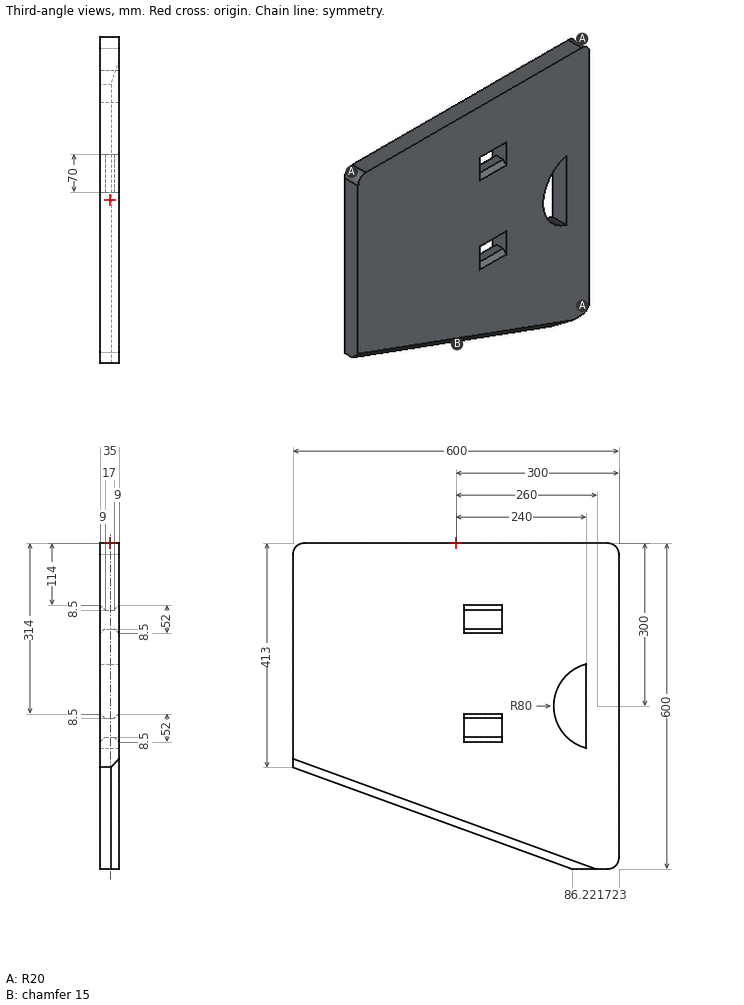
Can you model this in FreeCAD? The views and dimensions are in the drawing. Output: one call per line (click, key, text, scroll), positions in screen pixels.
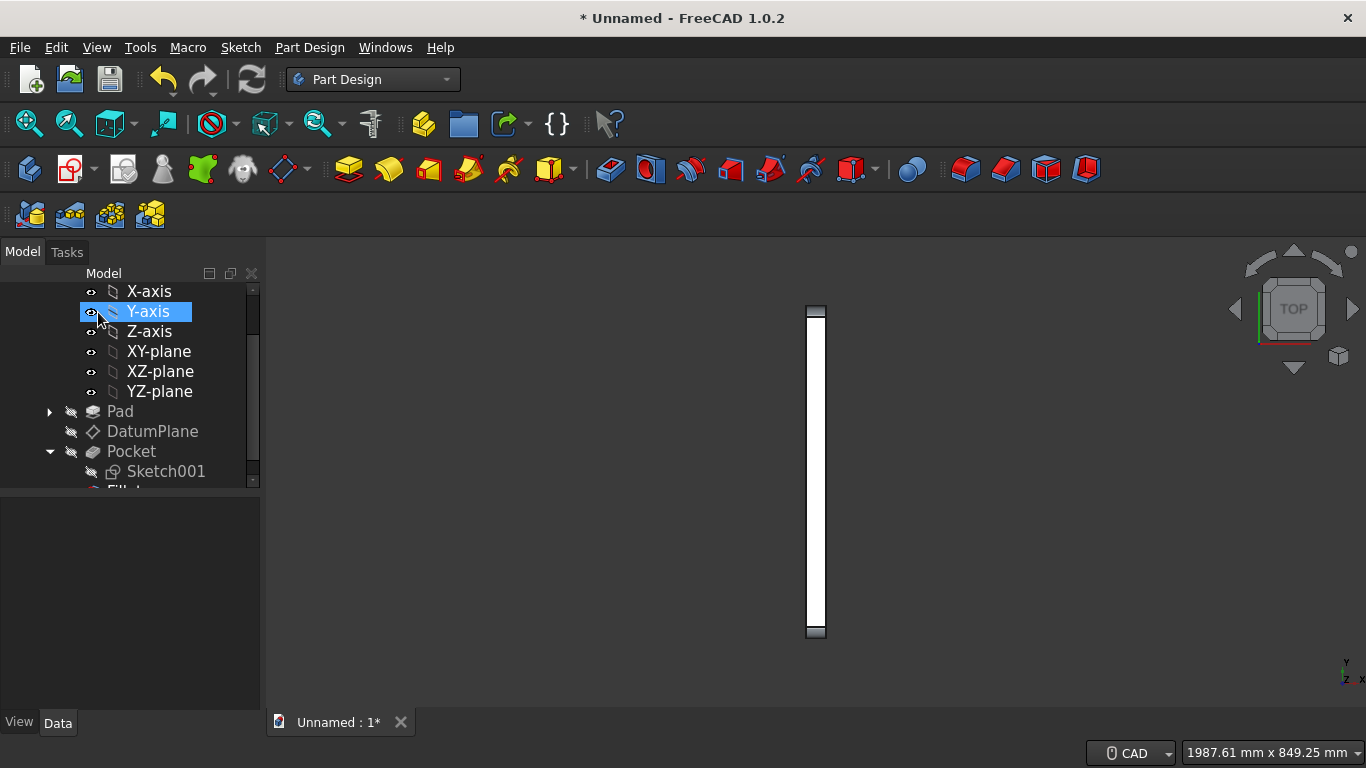
key(1)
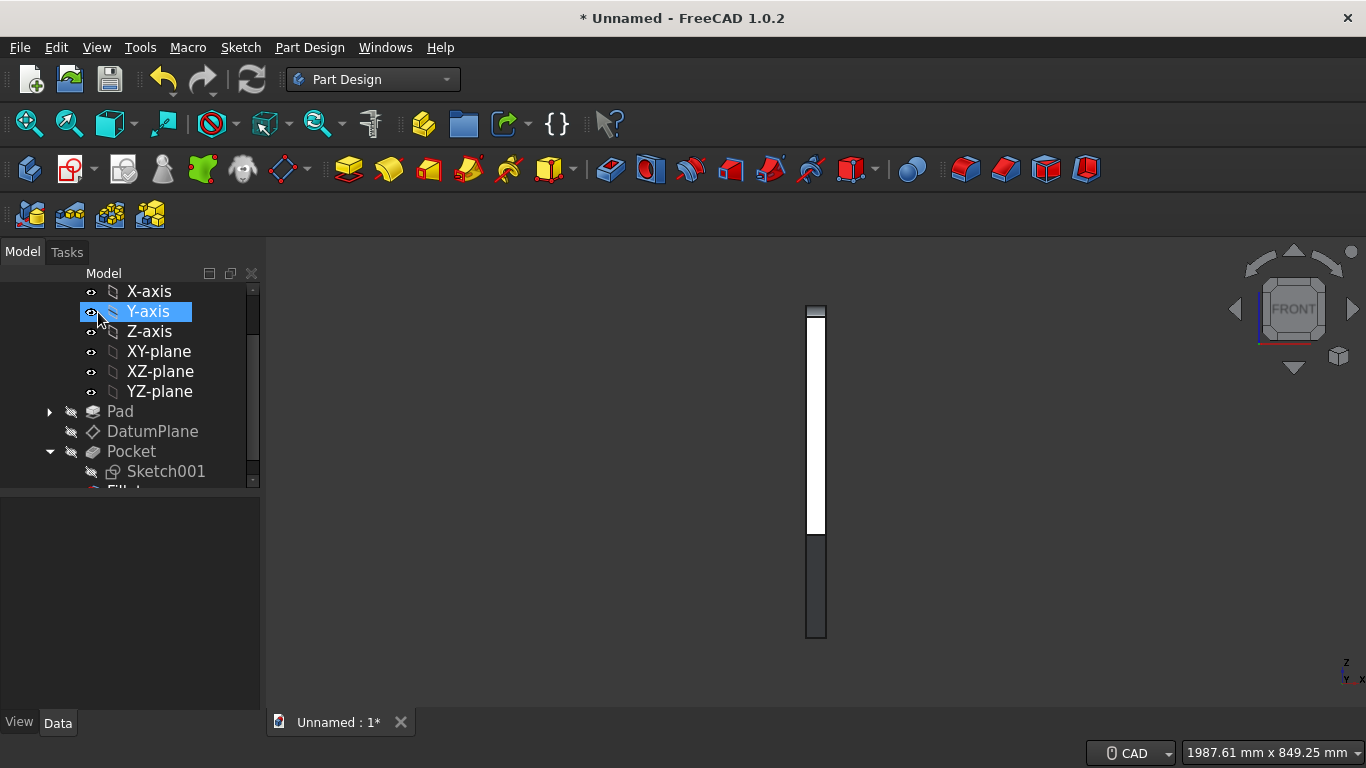
click(826, 585)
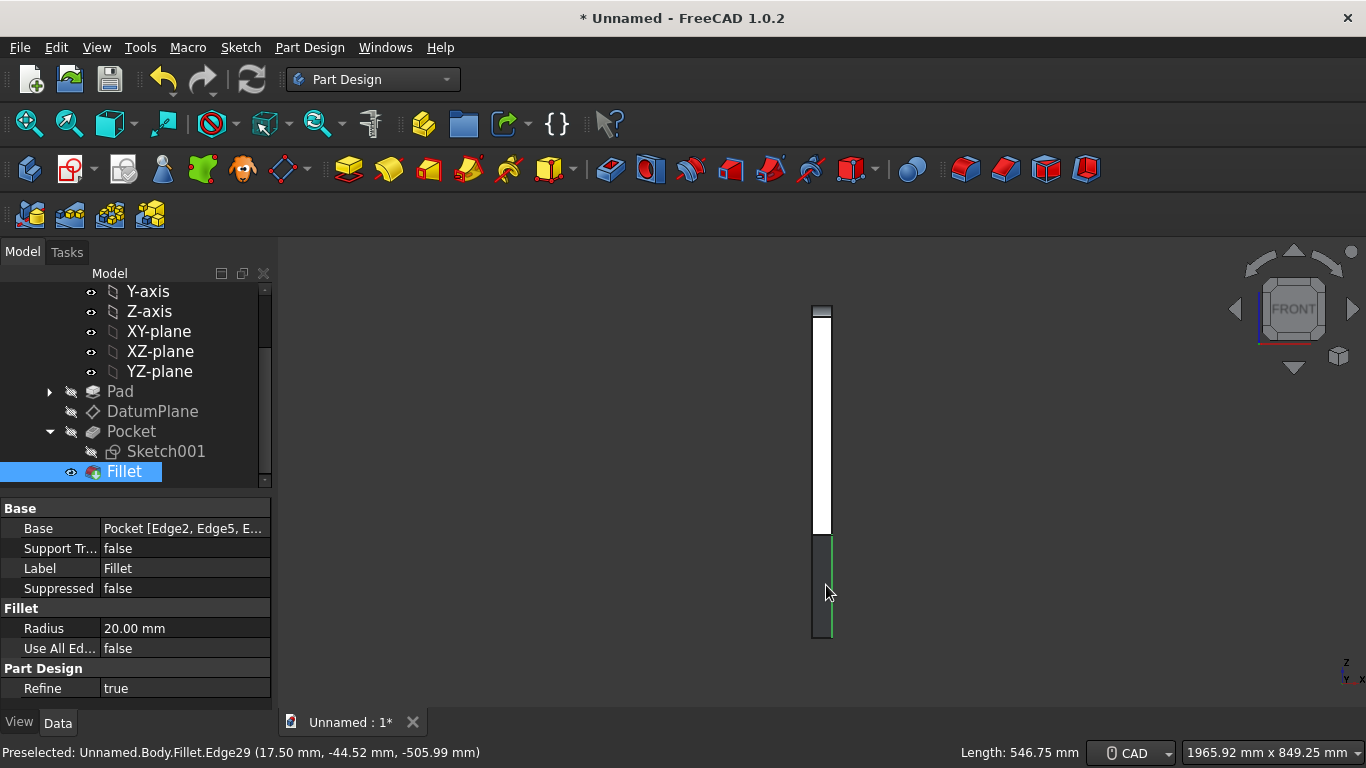
click(1006, 170)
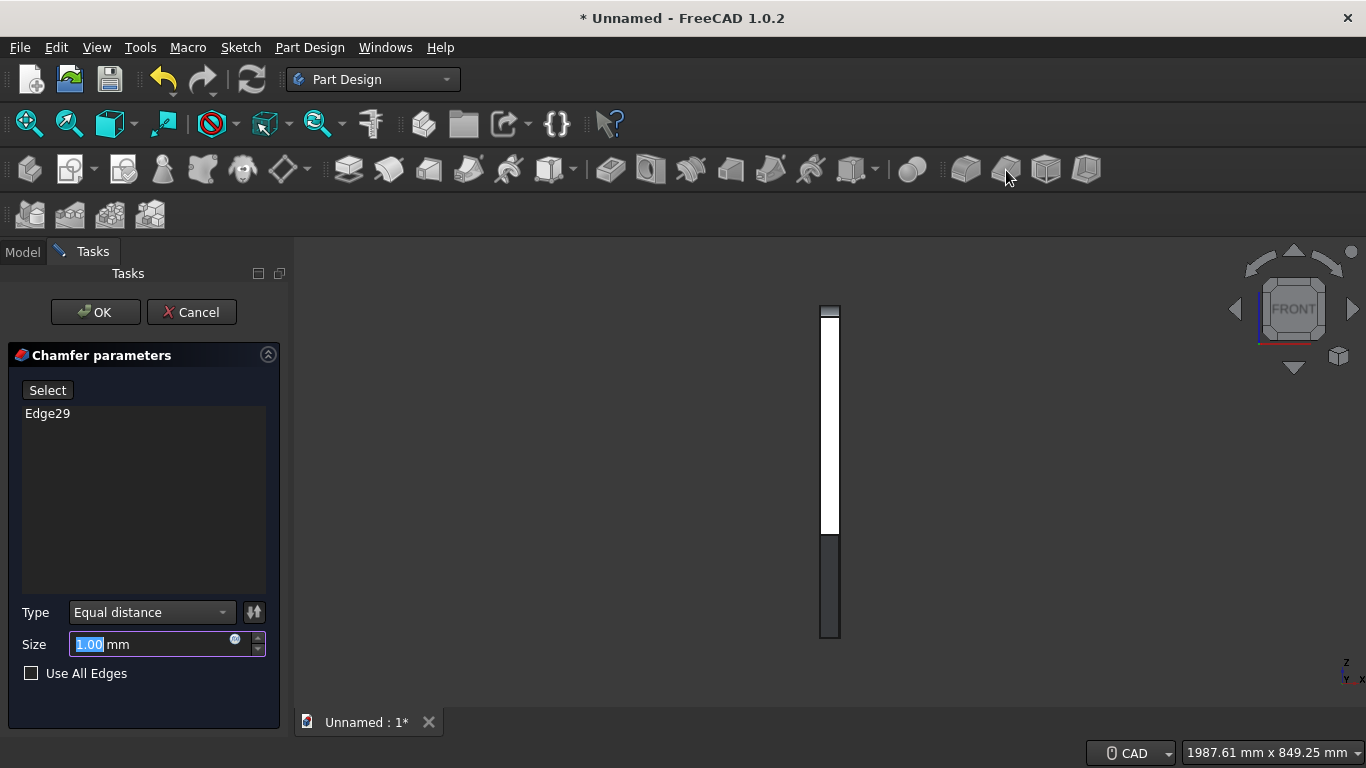
text(15)
key(Tab)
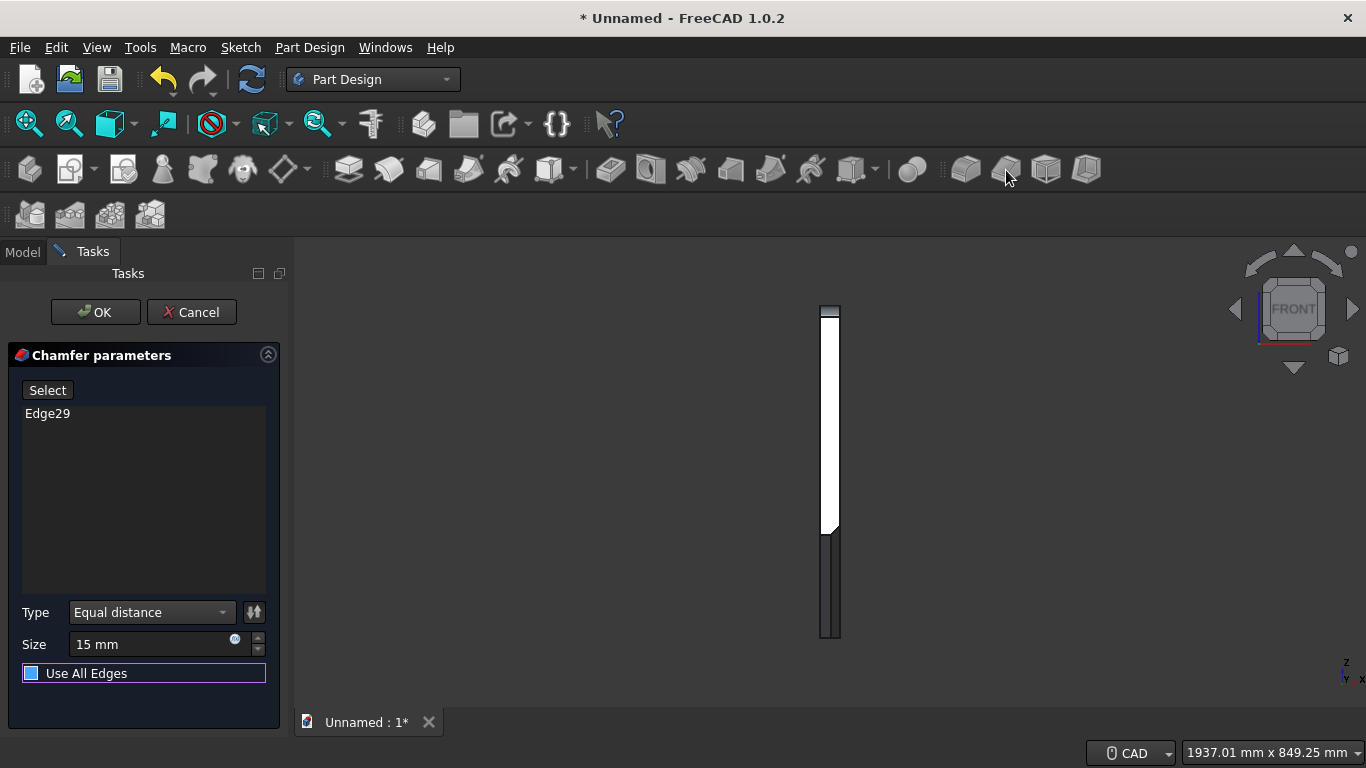
click(96, 312)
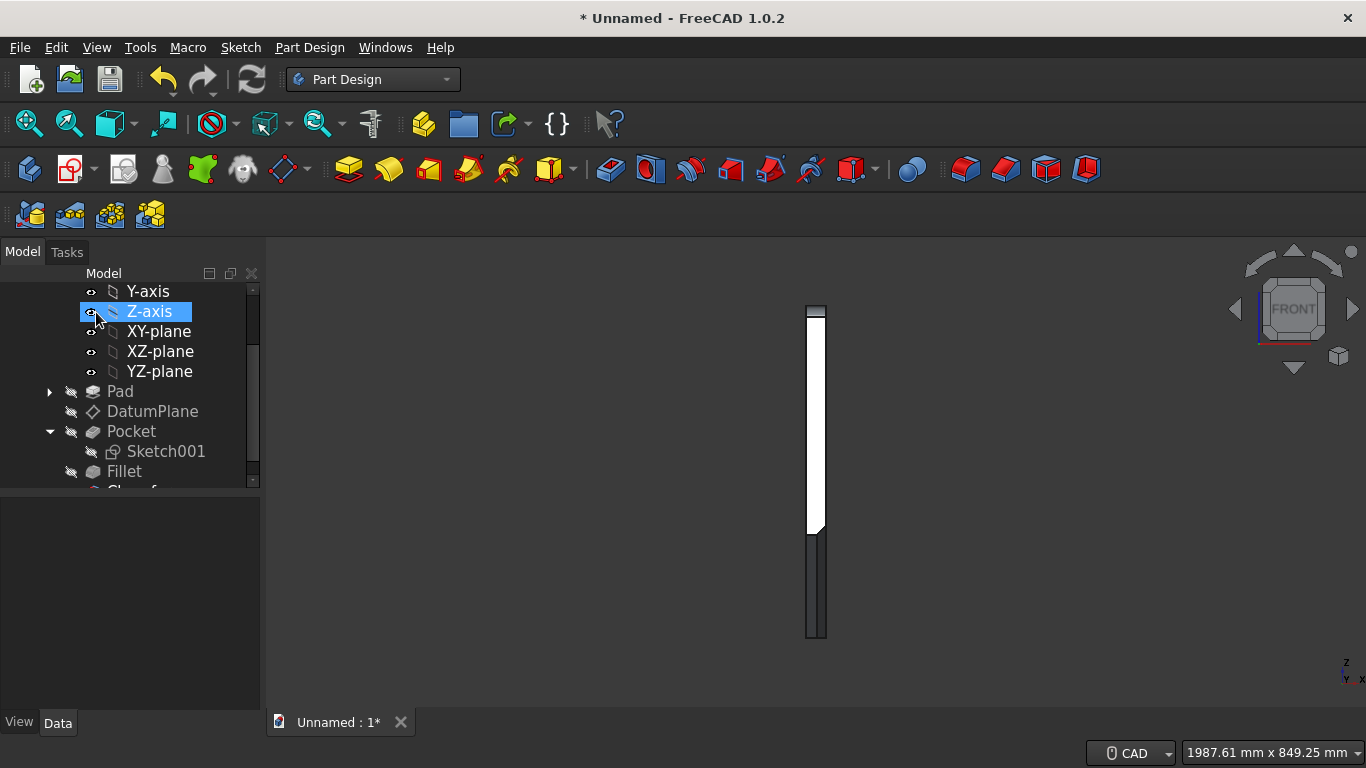
key(0)